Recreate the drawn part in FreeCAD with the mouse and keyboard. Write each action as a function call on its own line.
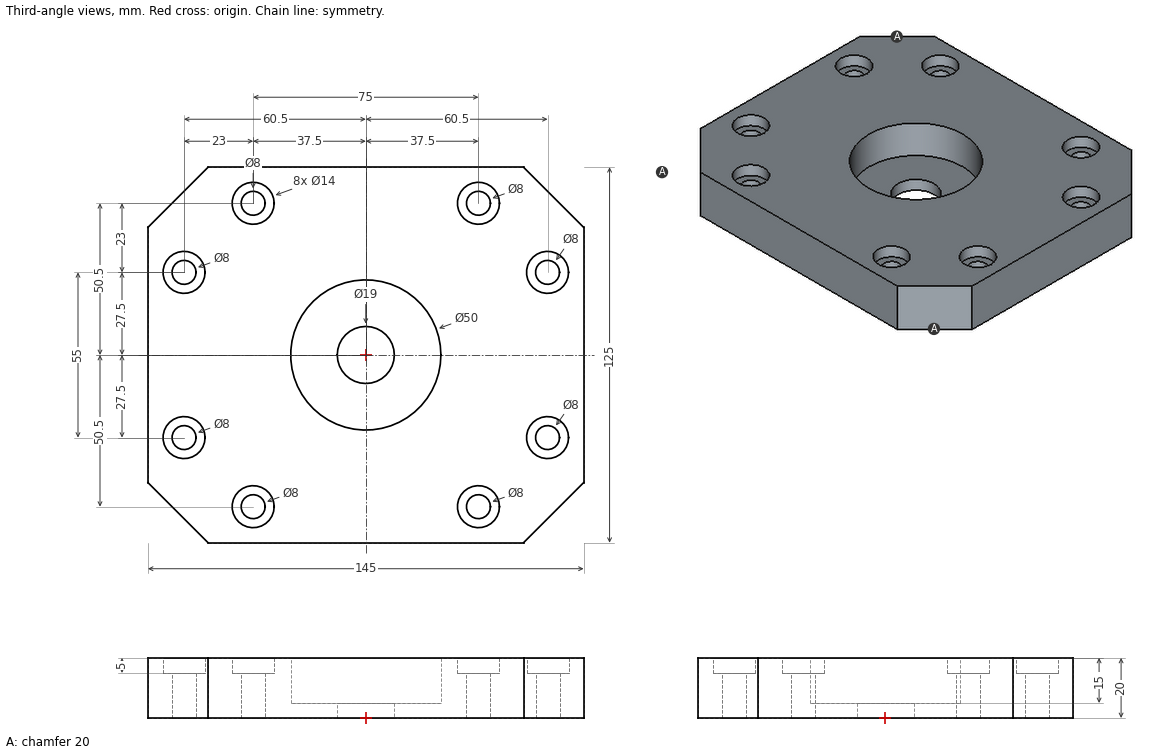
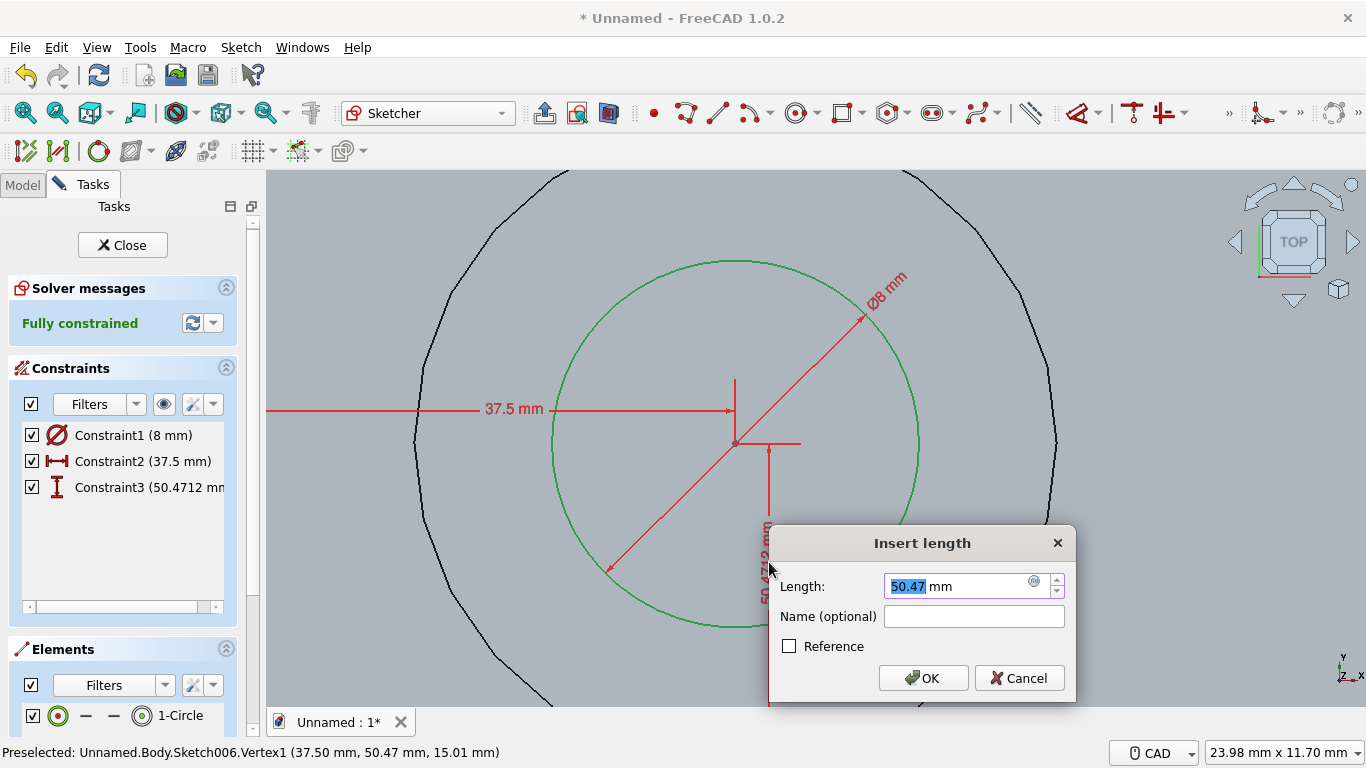
text(50.5)
key(Return)
key(Escape)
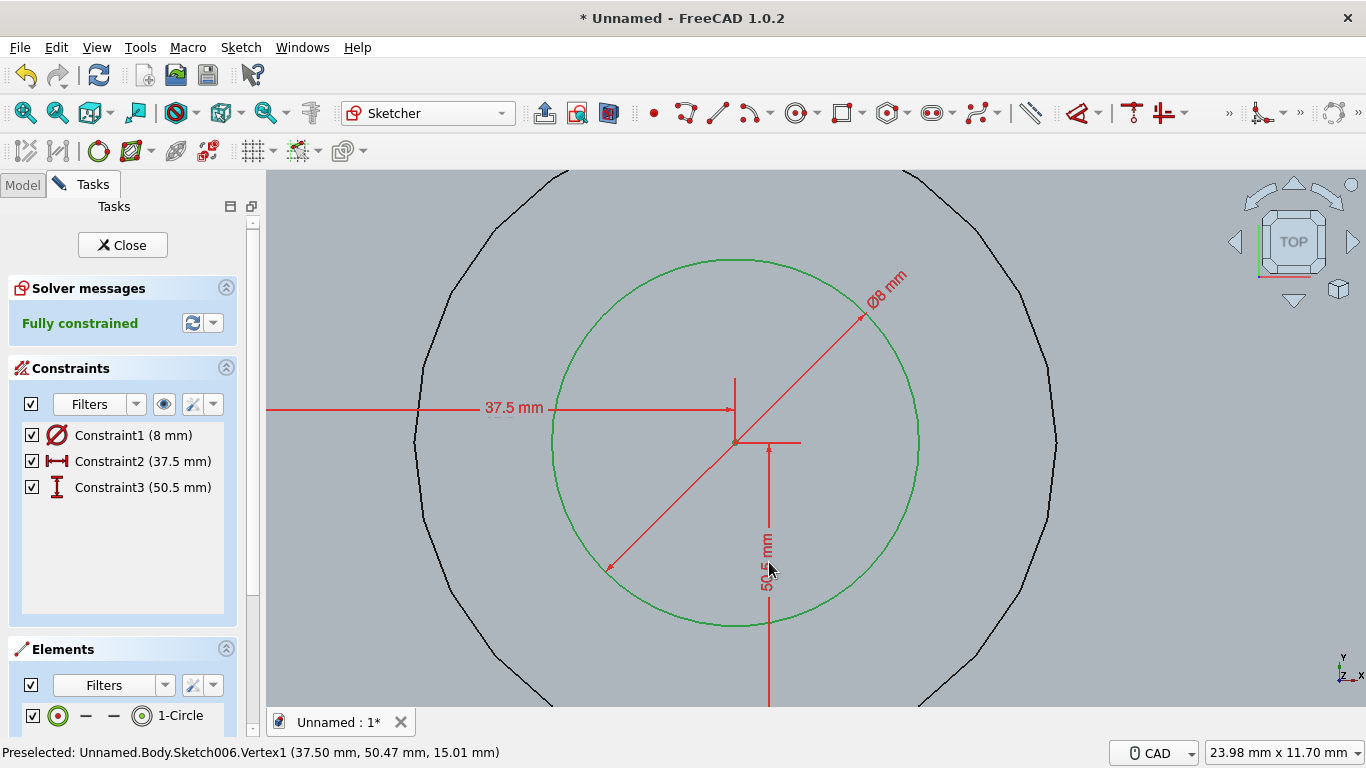
click(123, 245)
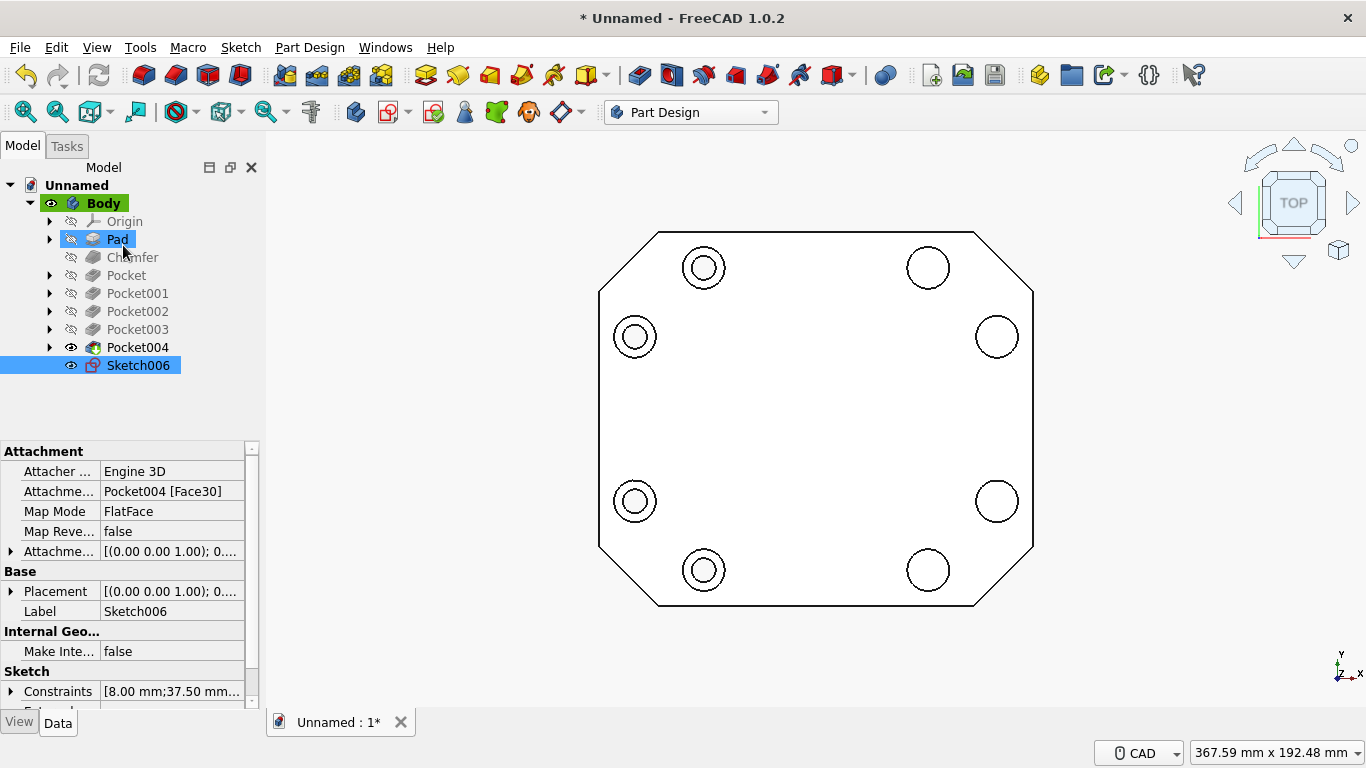
click(640, 76)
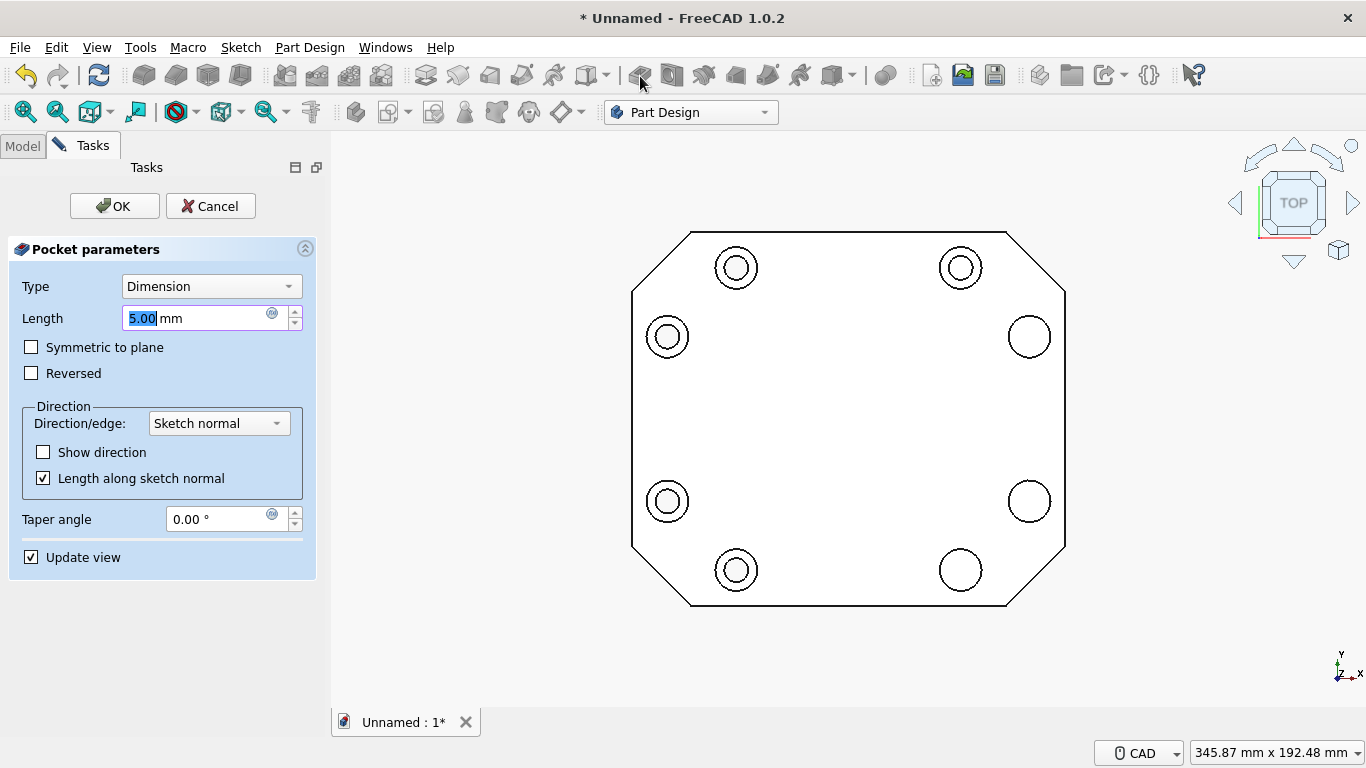
click(212, 286)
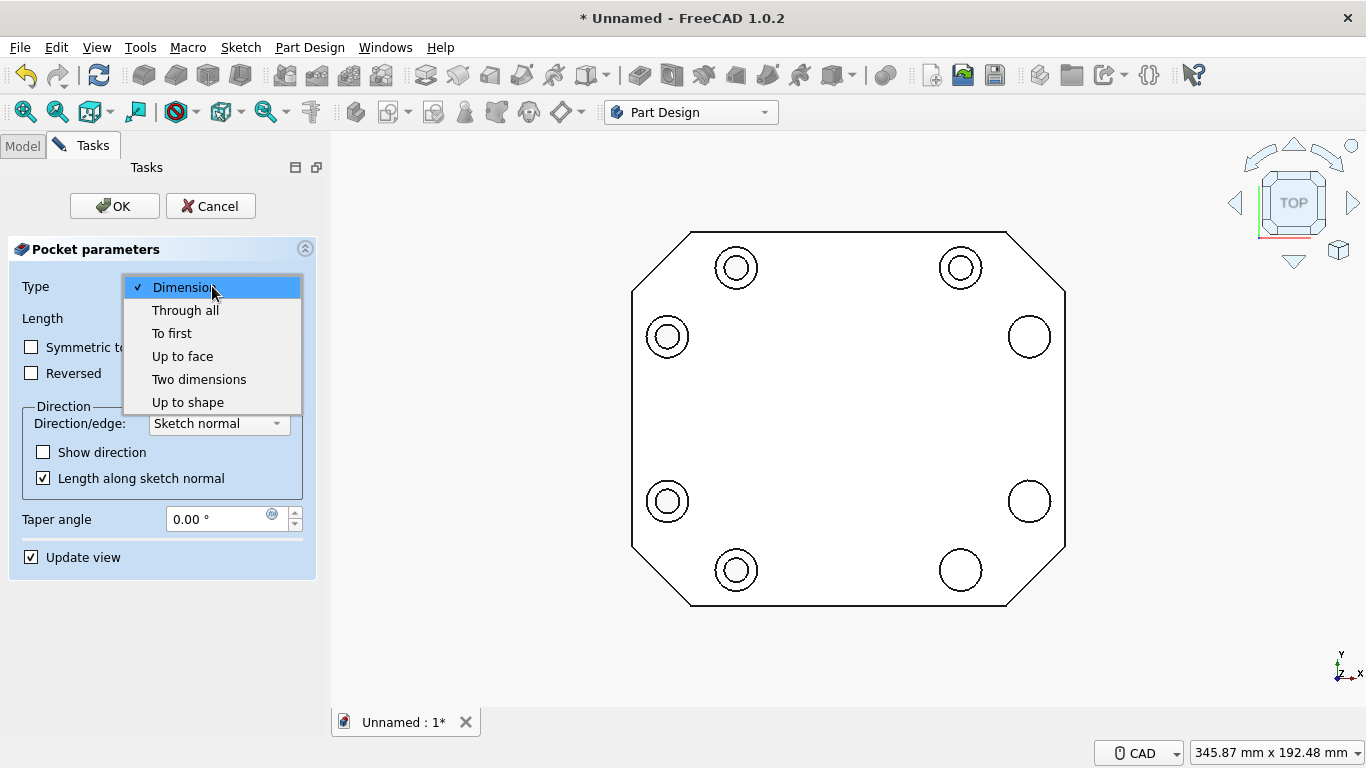
click(212, 334)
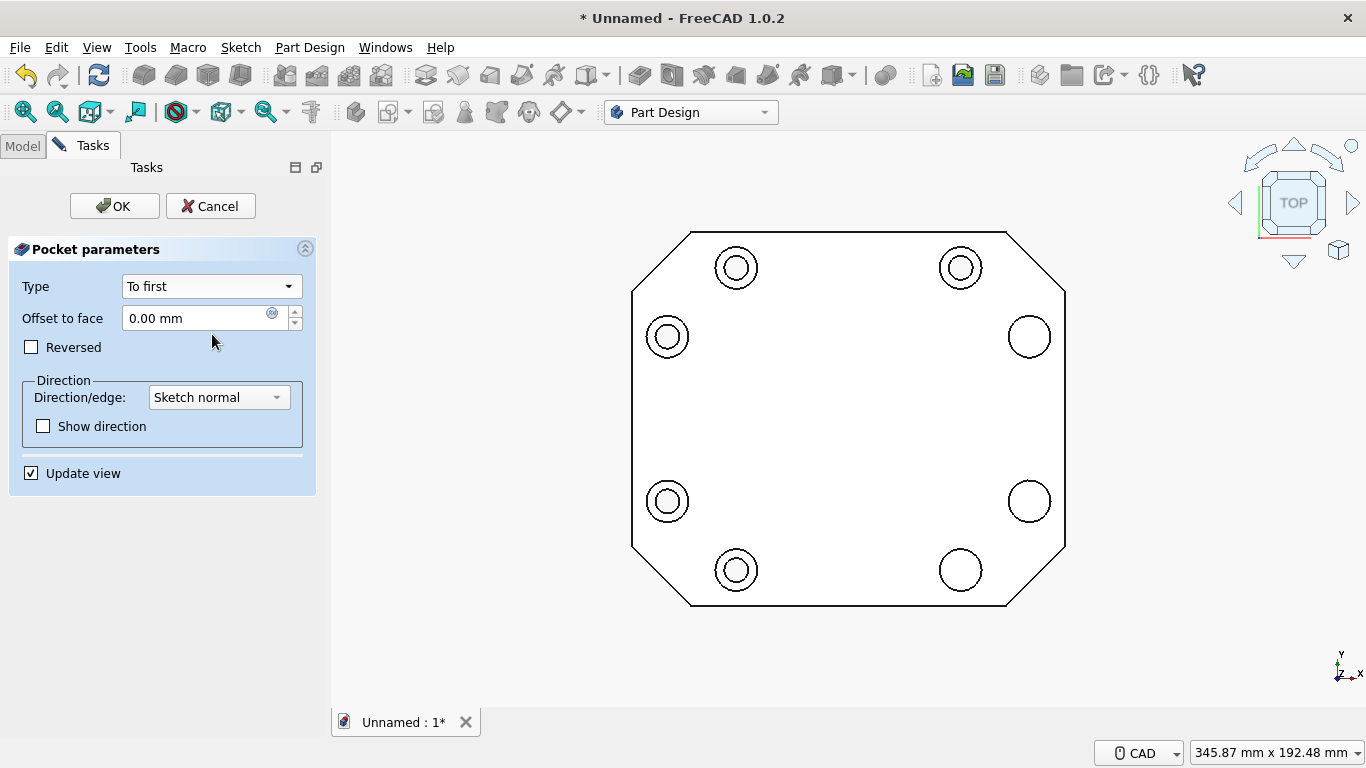
click(115, 206)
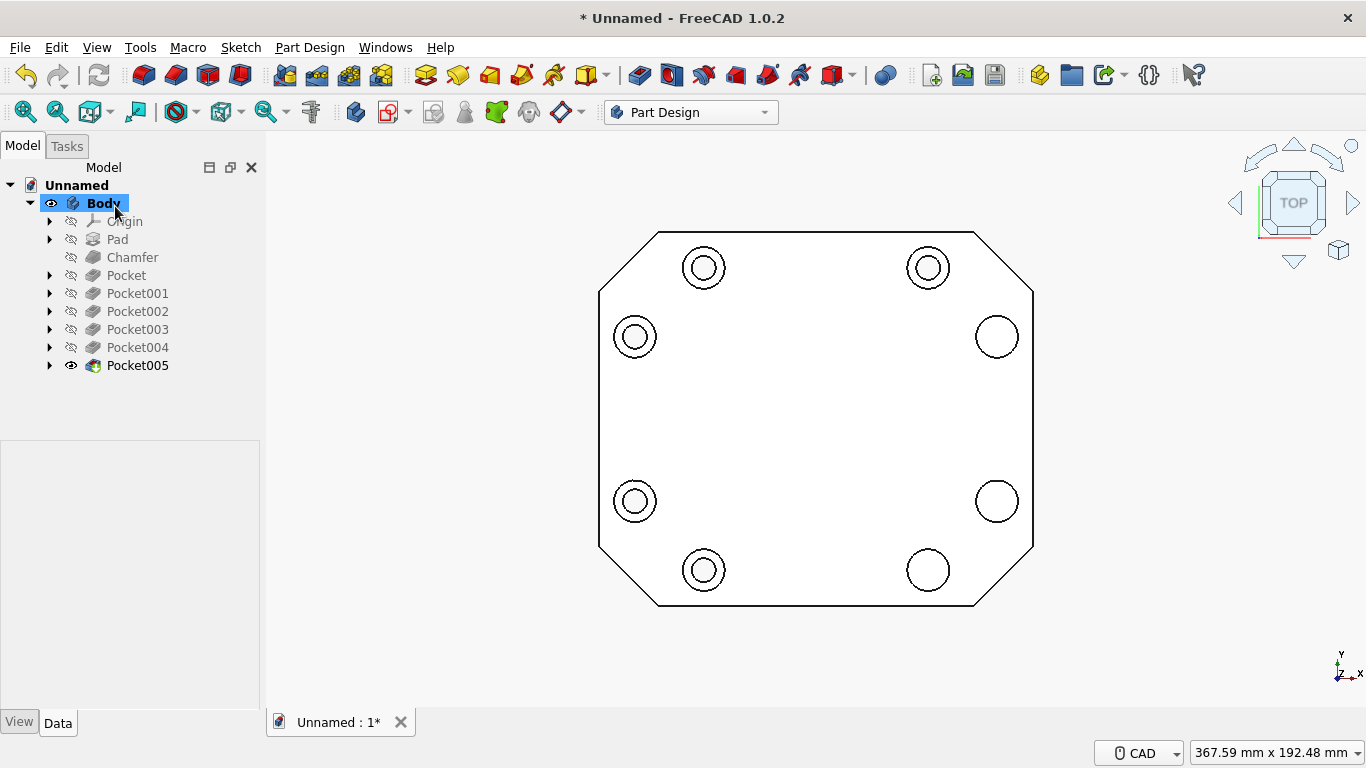
click(928, 569)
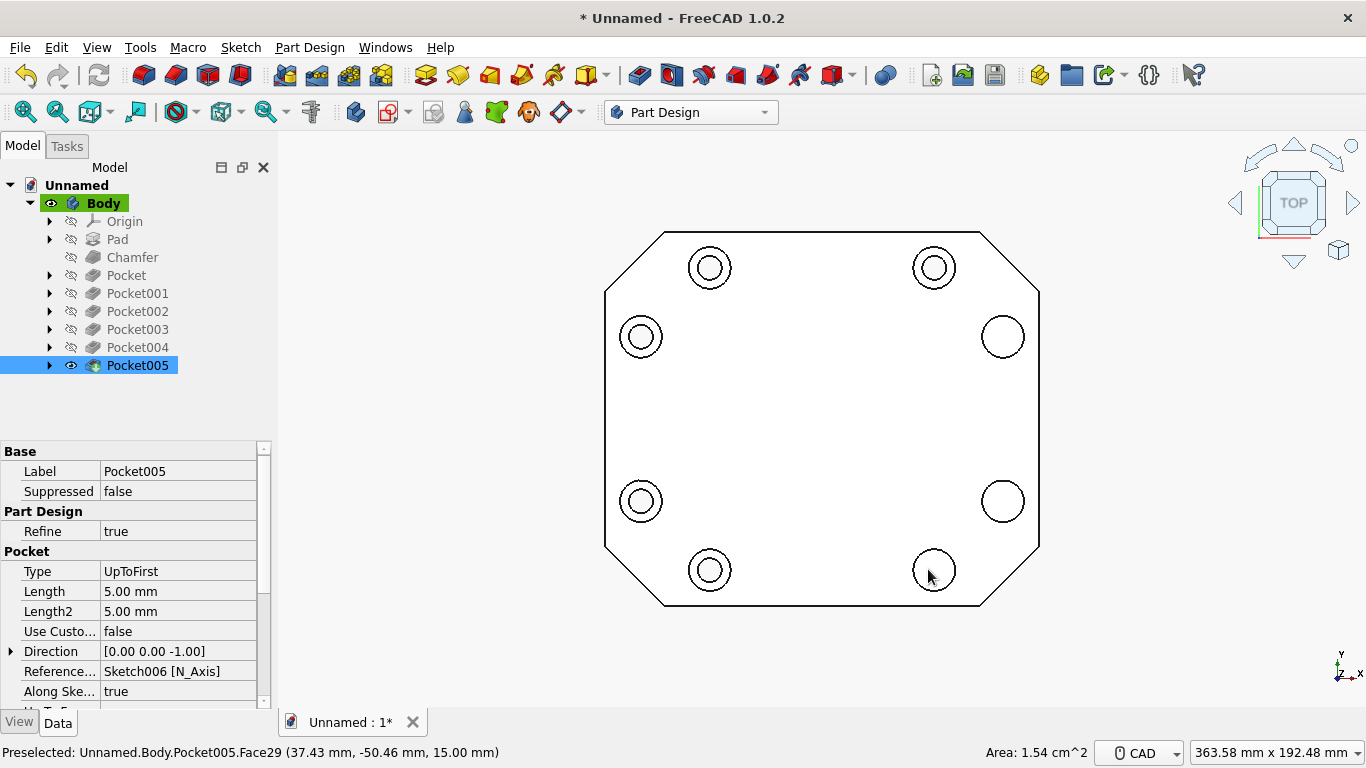
click(388, 112)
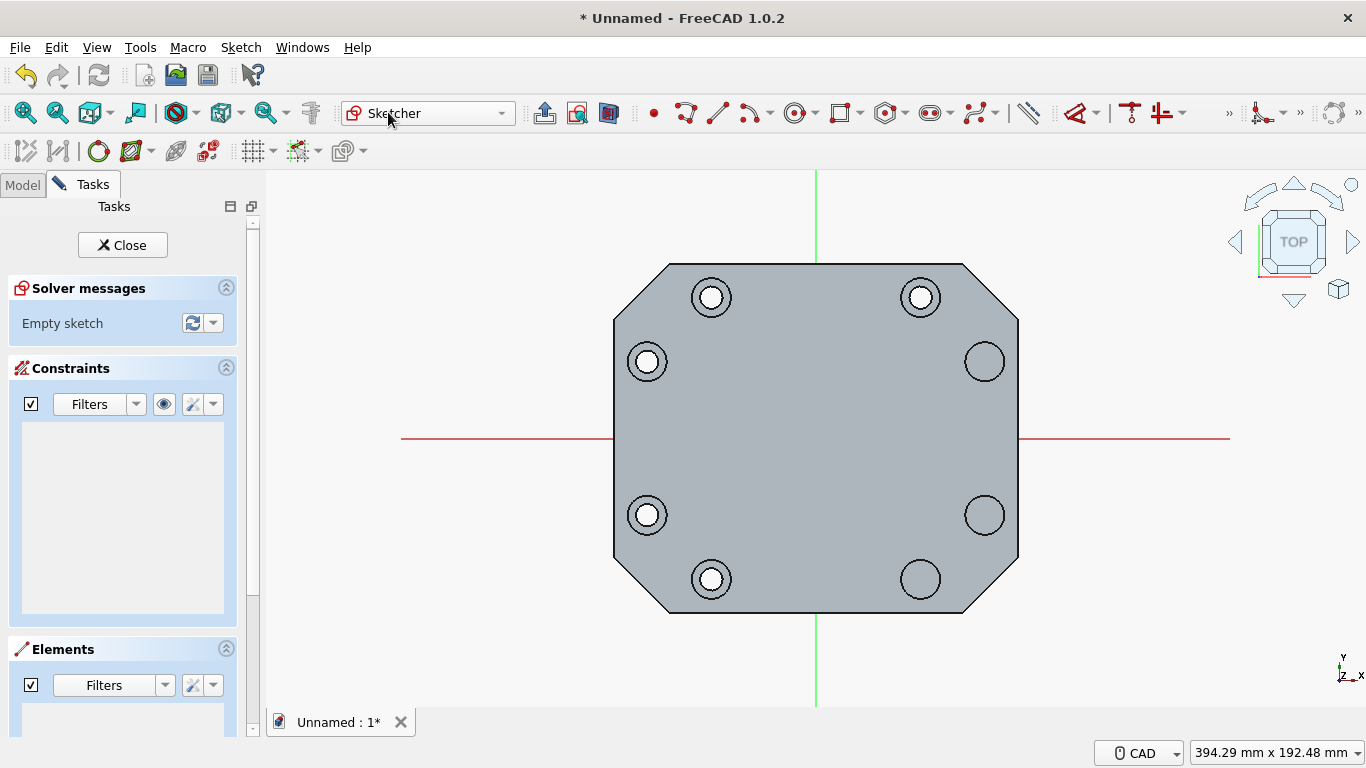
scroll(1000, 357, up, 14)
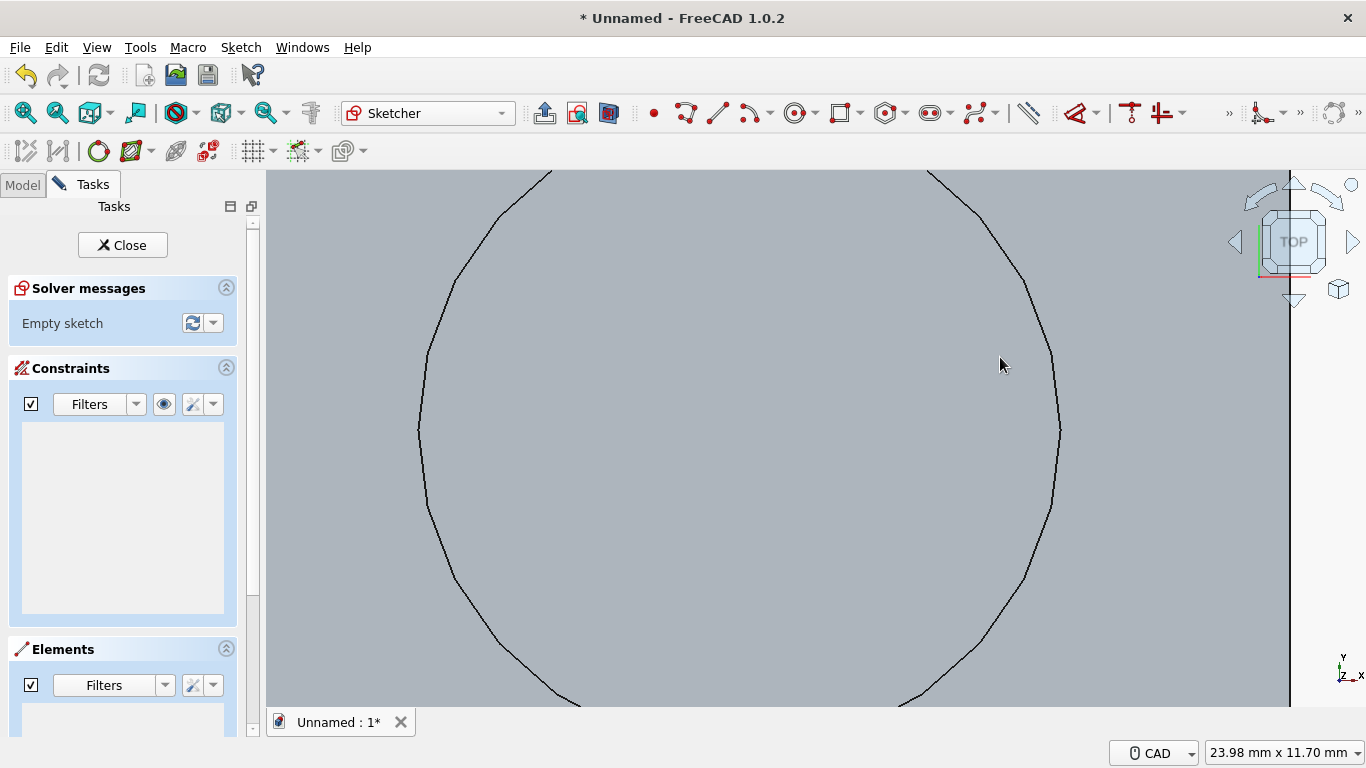
click(796, 114)